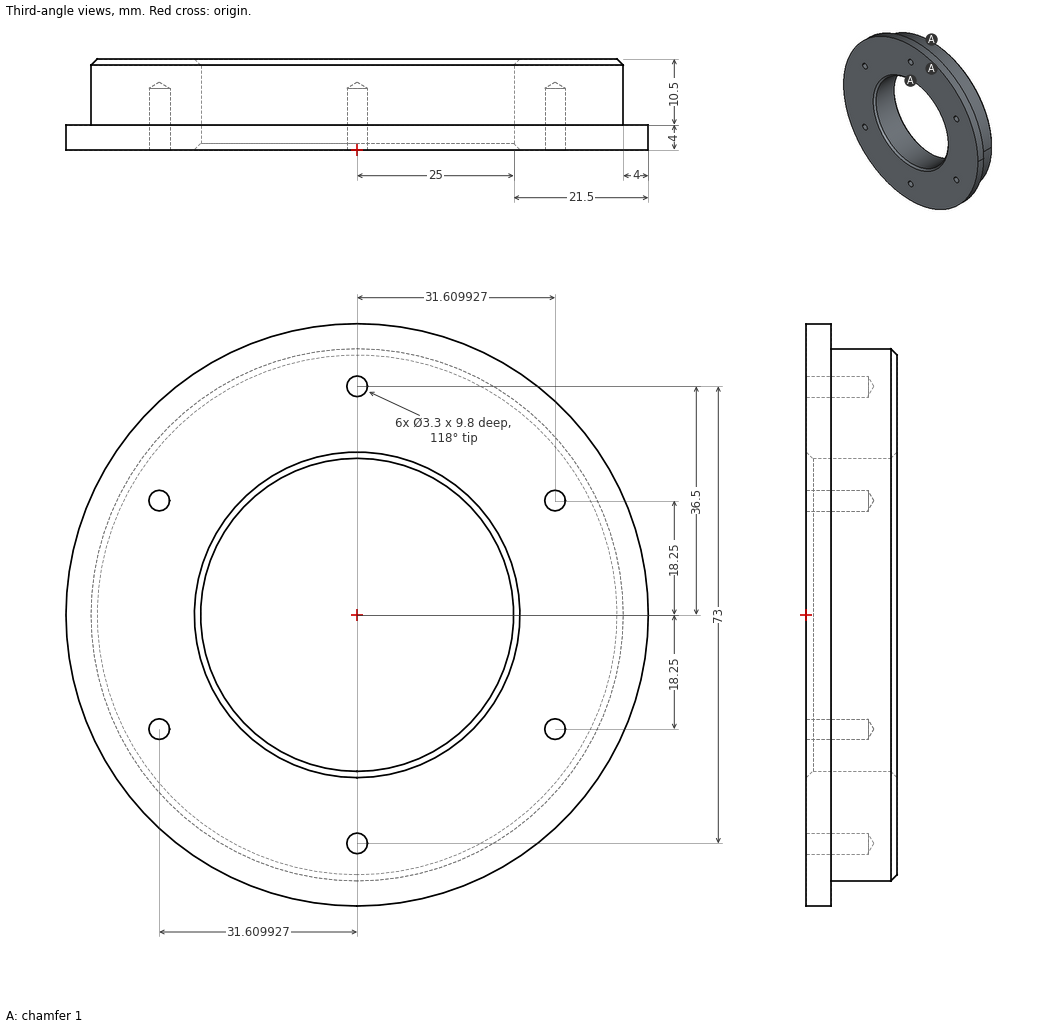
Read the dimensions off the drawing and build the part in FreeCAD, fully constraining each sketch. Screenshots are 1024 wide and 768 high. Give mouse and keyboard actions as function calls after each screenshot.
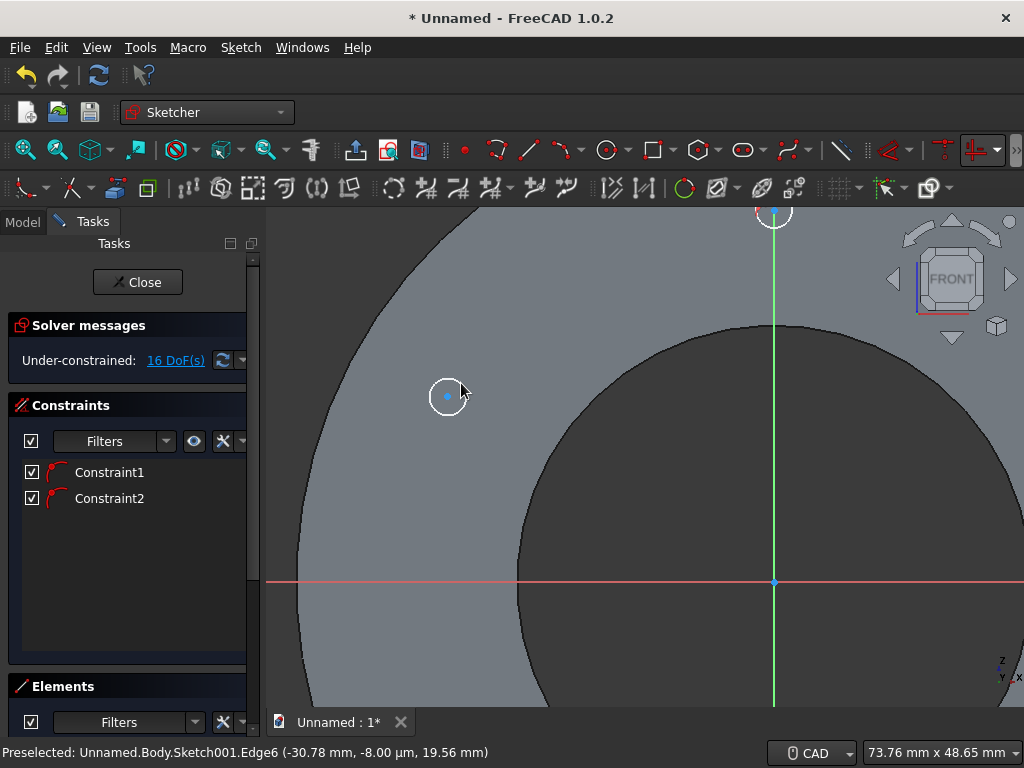
scroll(462, 384, down, 5)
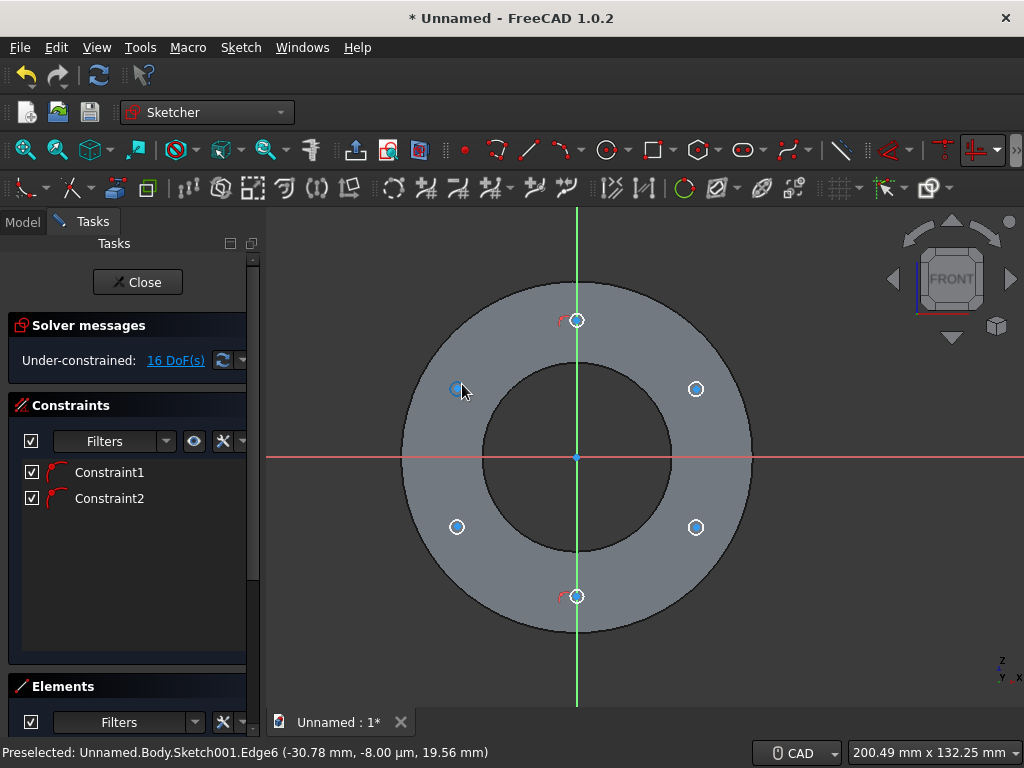
scroll(582, 316, up, 6)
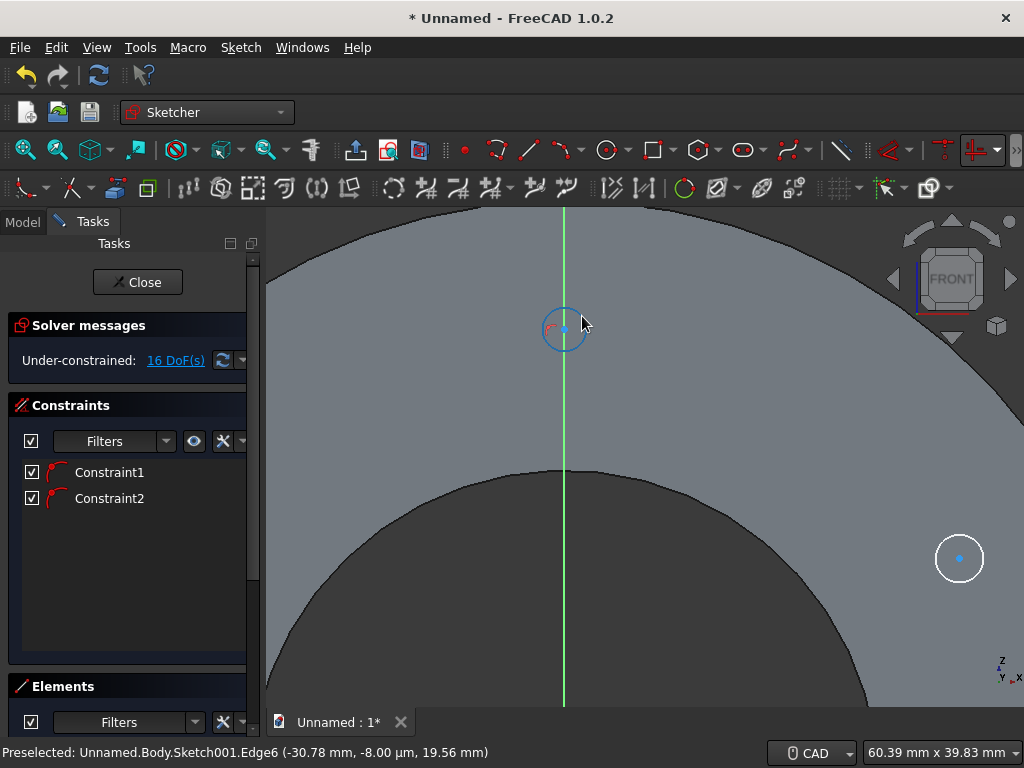
click(580, 314)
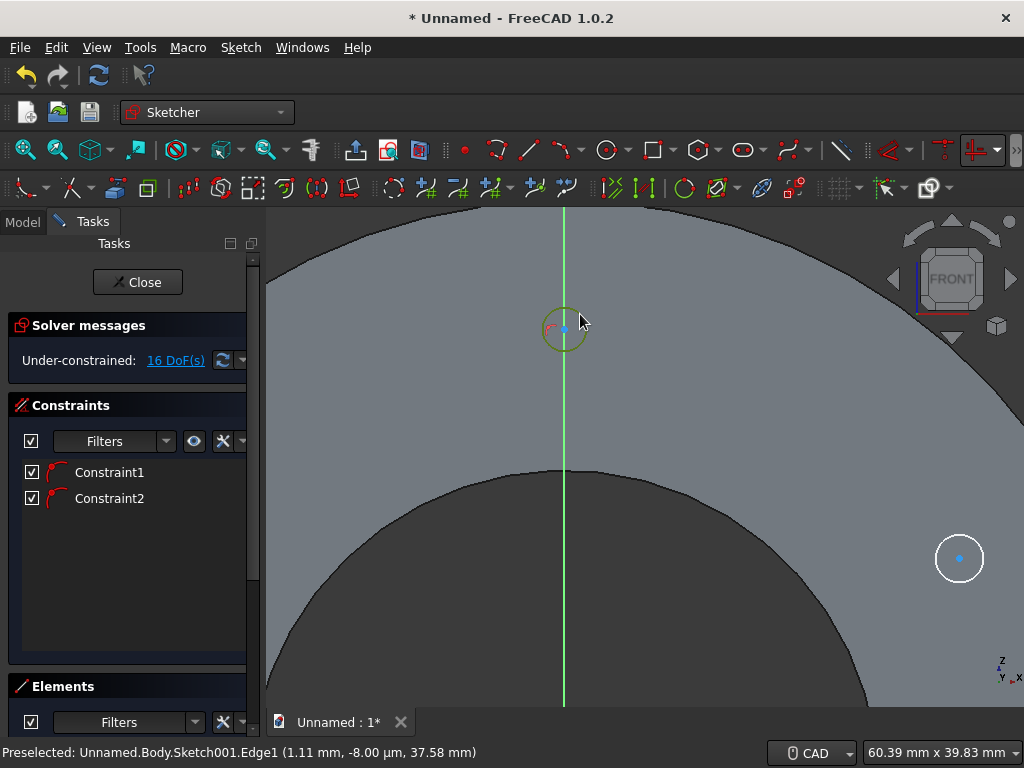
scroll(582, 316, down, 6)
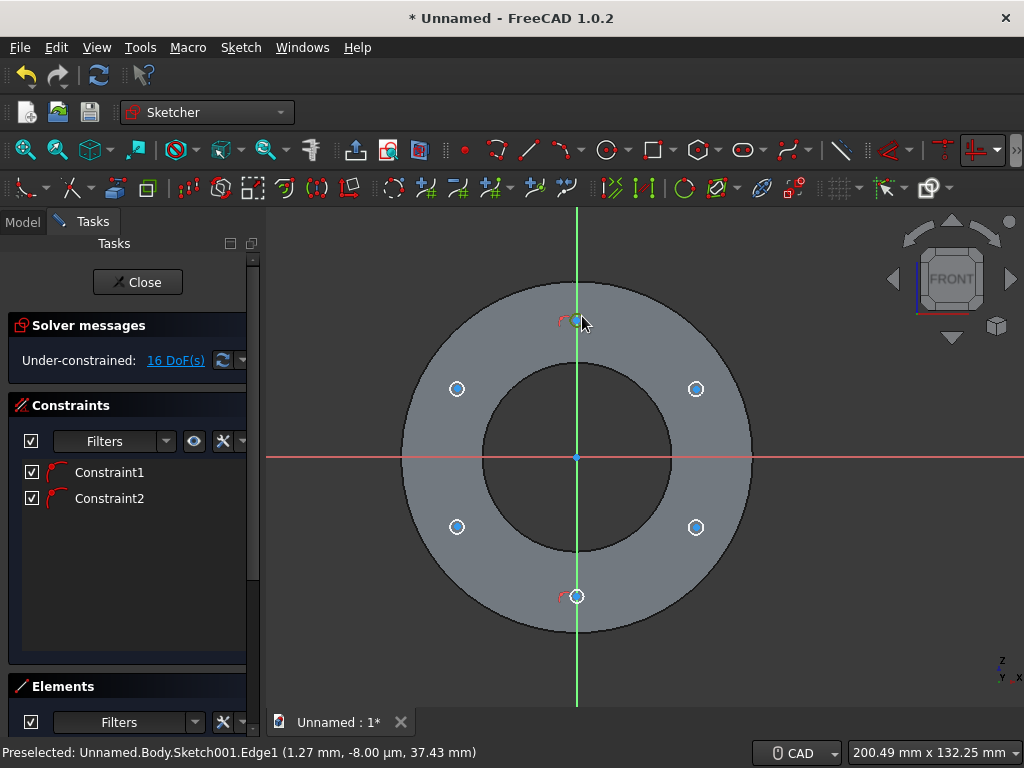
scroll(701, 384, up, 4)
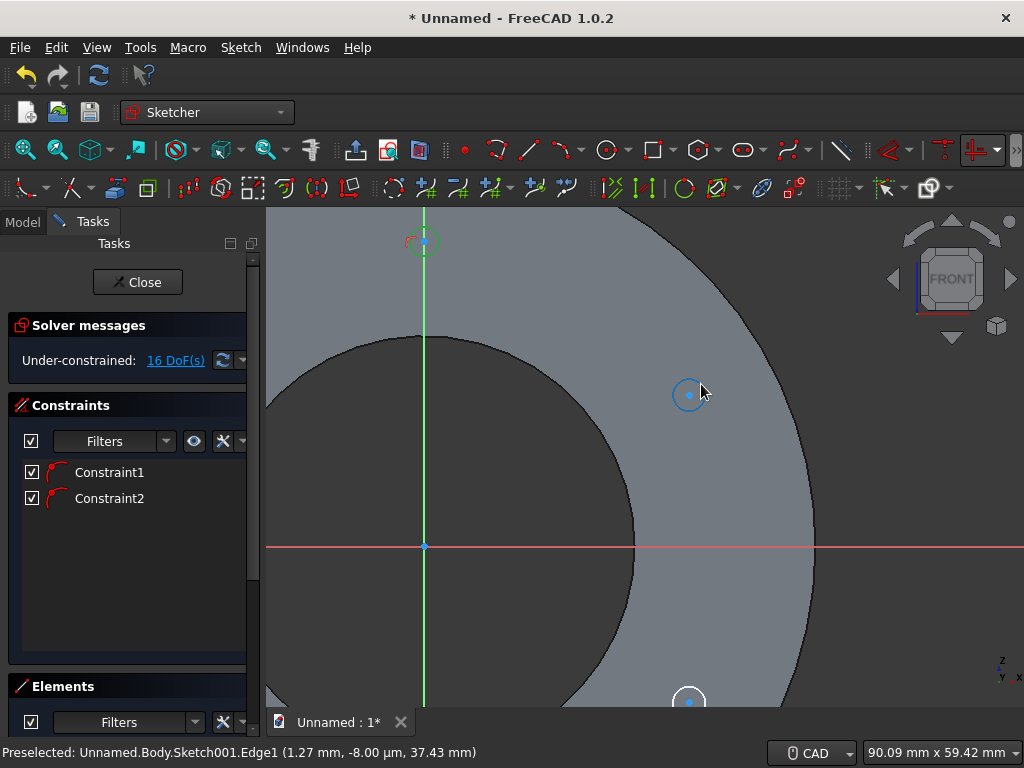
click(700, 384)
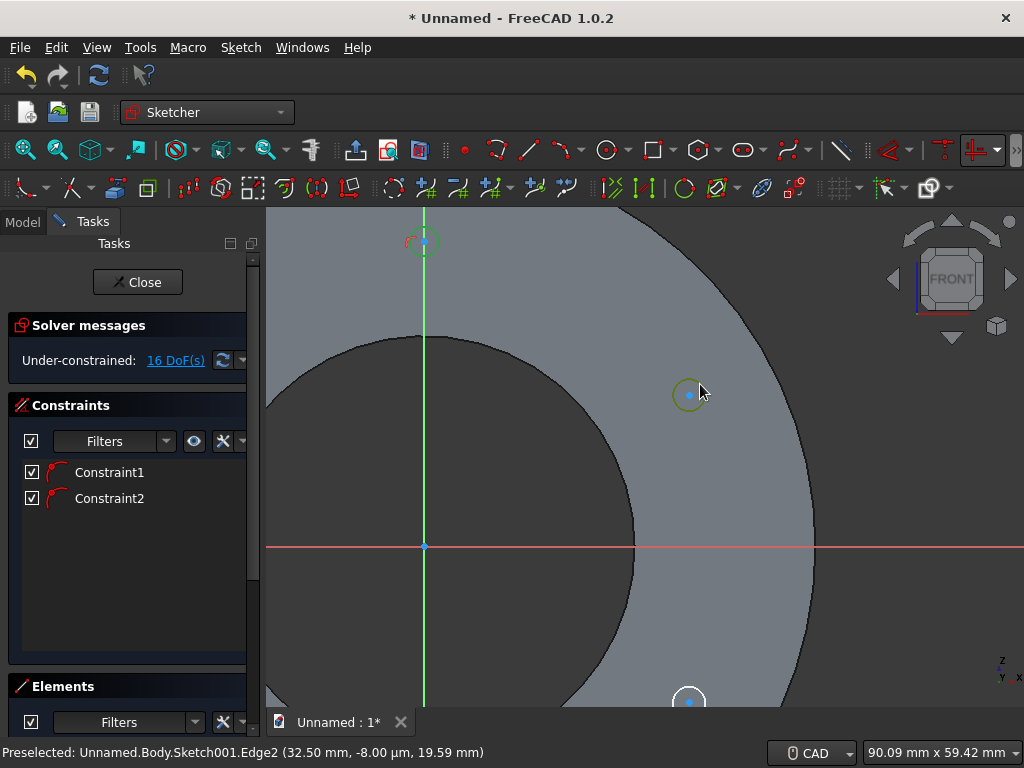
scroll(701, 384, down, 4)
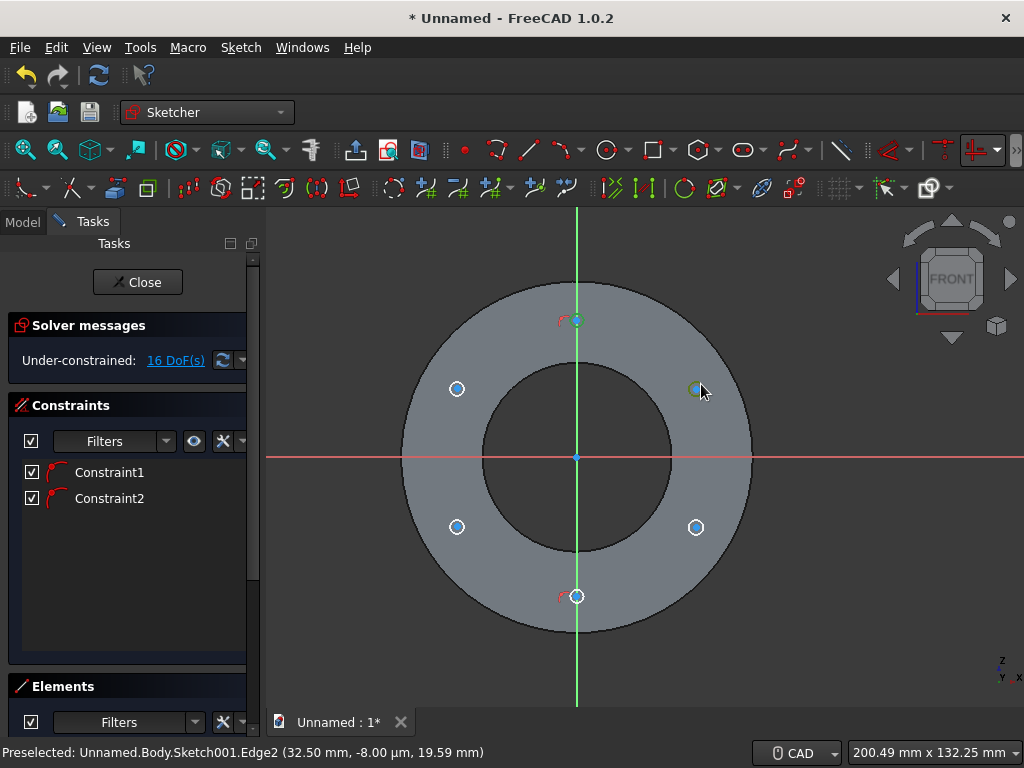
scroll(701, 522, up, 4)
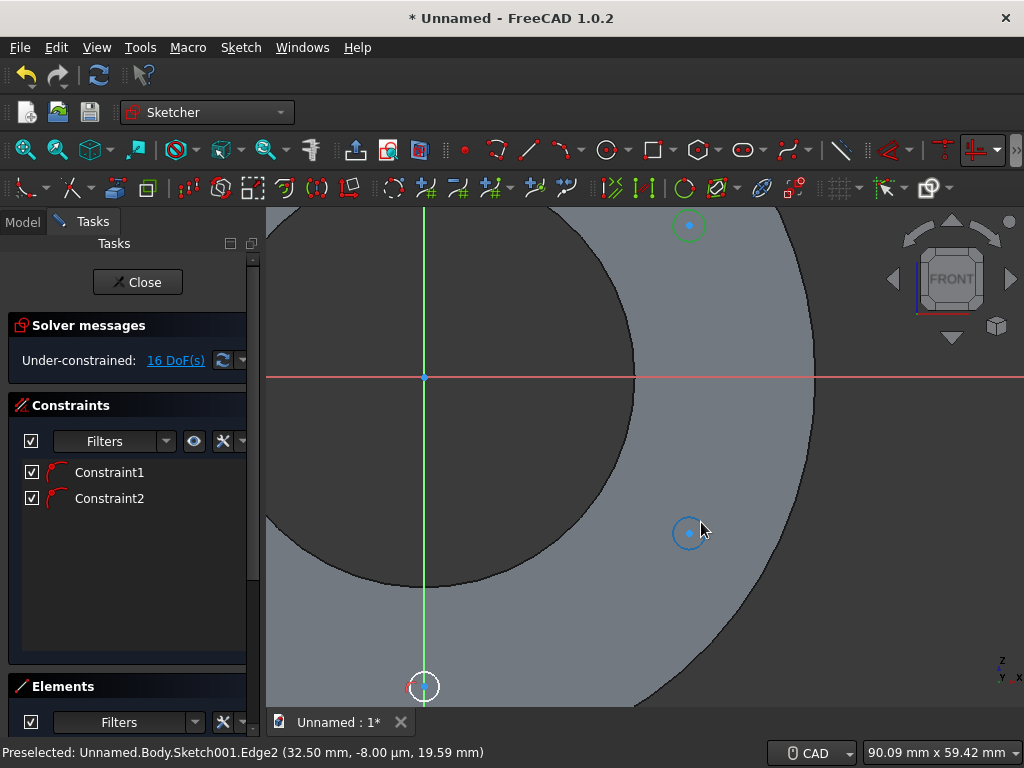
click(701, 522)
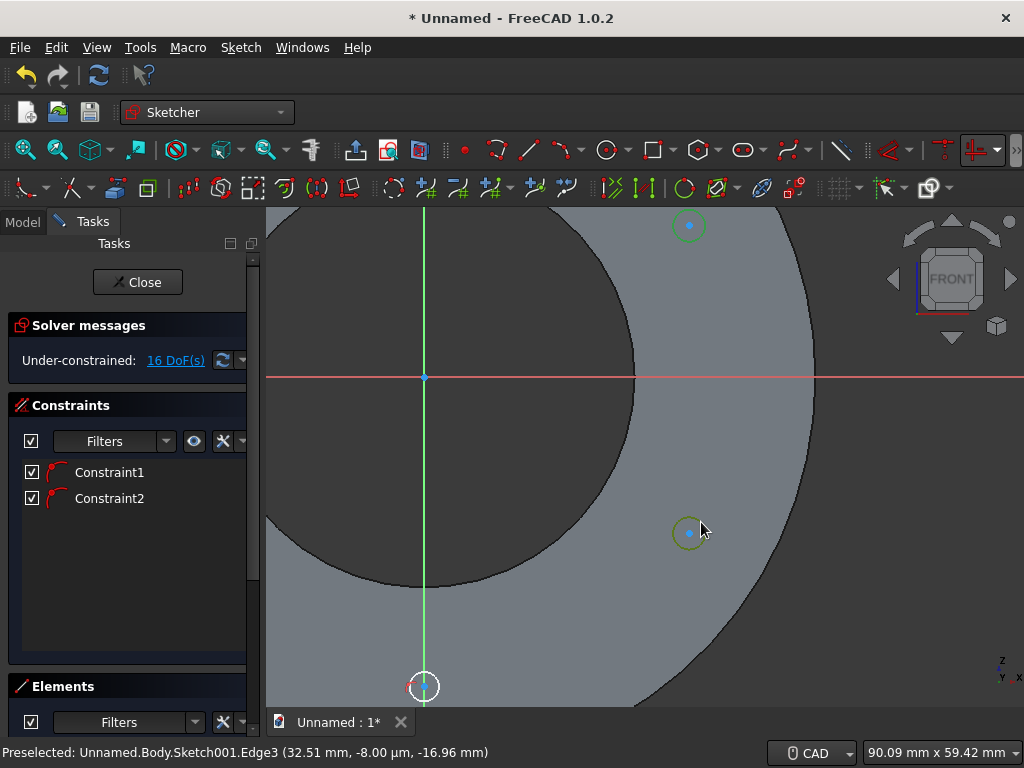
scroll(435, 676, up, 2)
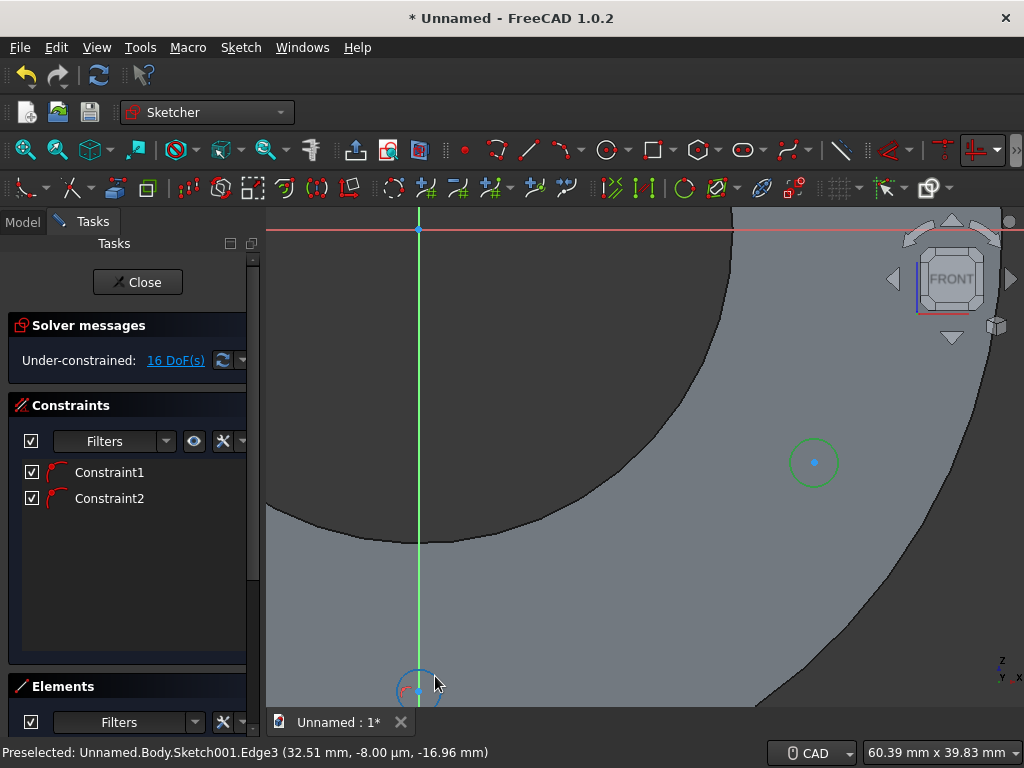
click(434, 676)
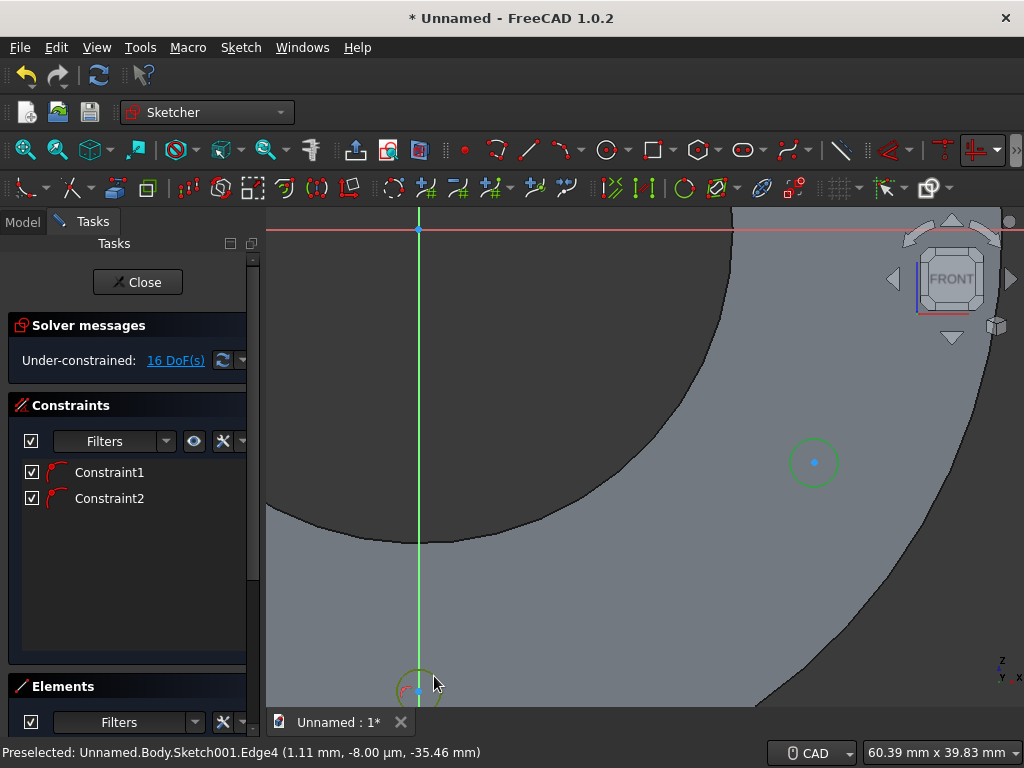
scroll(644, 555, down, 6)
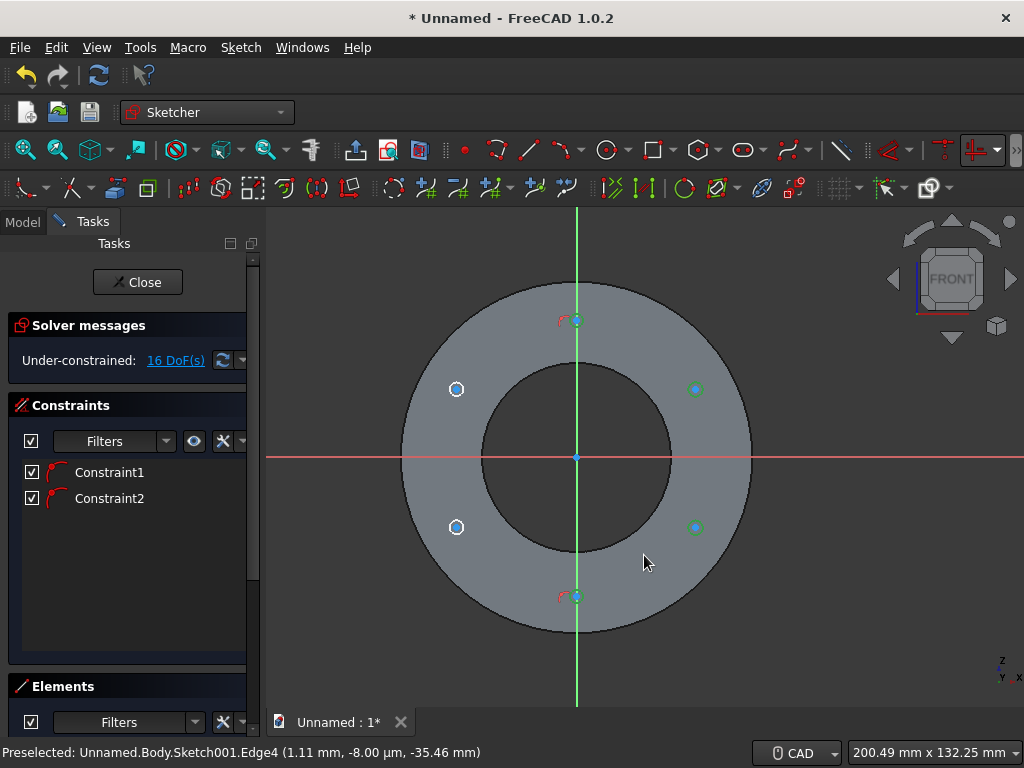
scroll(461, 522, up, 4)